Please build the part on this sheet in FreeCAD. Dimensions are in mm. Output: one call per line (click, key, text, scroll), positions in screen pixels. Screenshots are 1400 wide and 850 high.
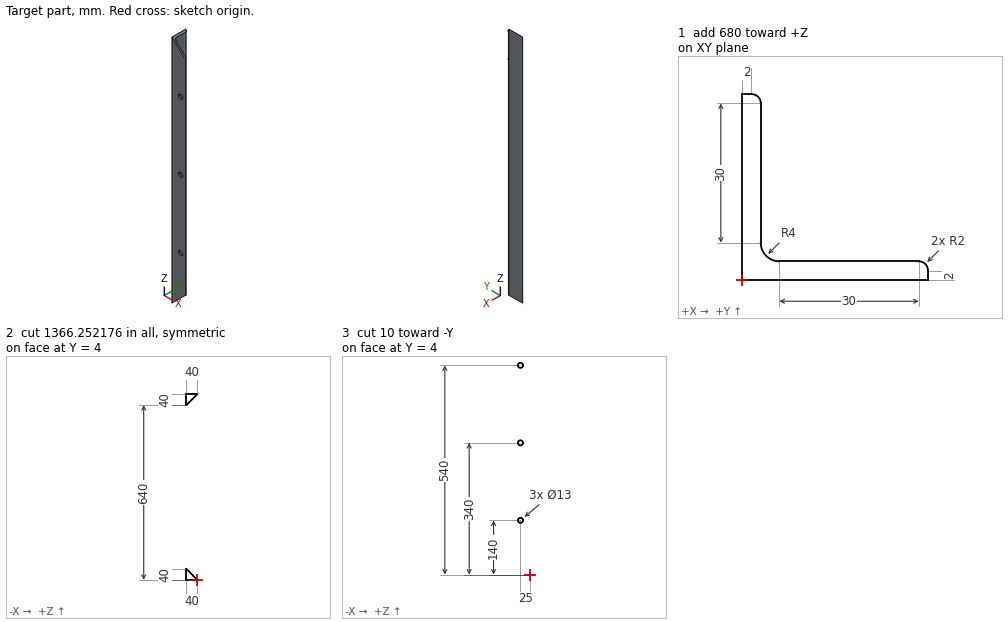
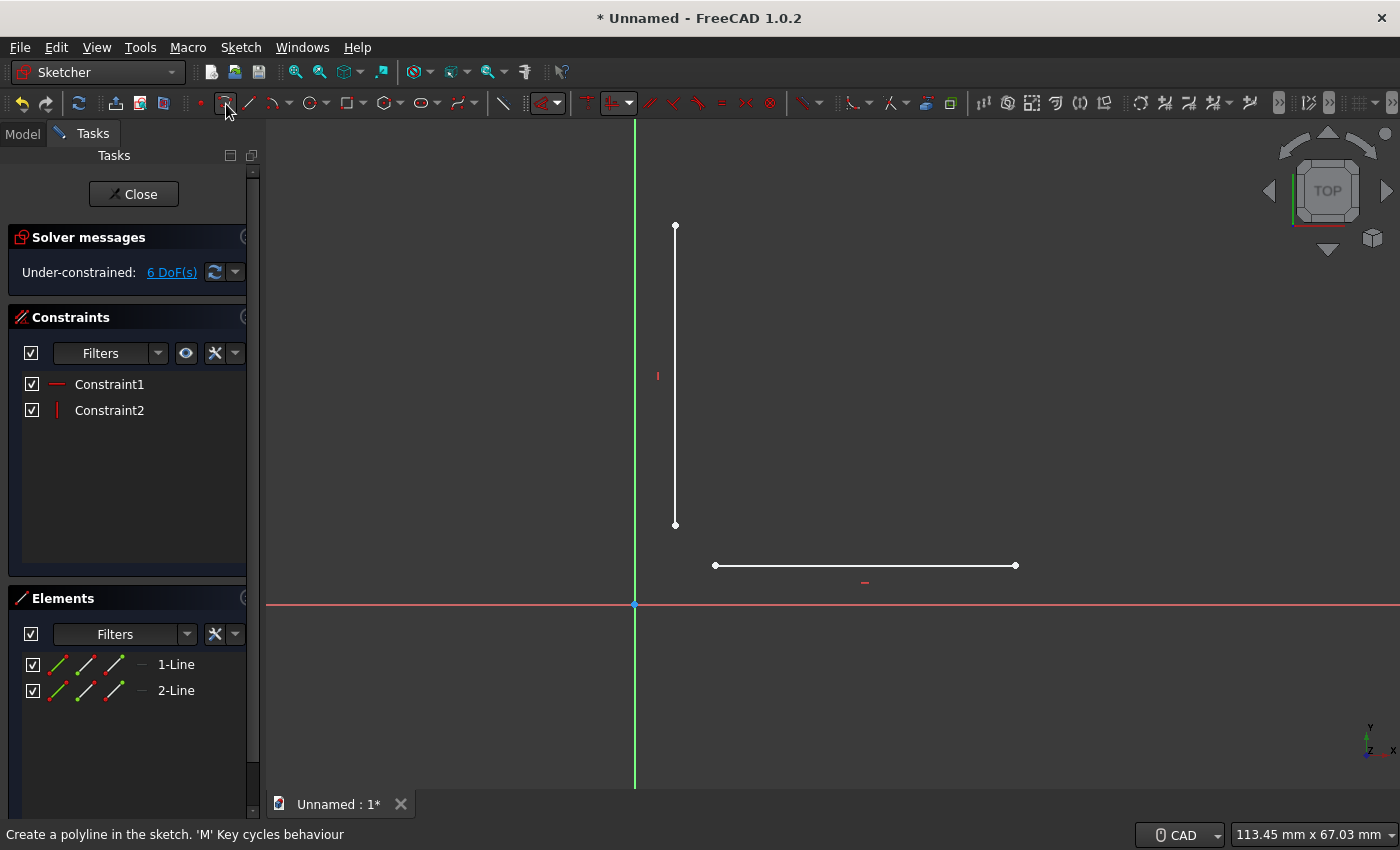
click(655, 205)
click(635, 205)
click(635, 605)
click(1035, 596)
click(1035, 585)
right_click(1035, 585)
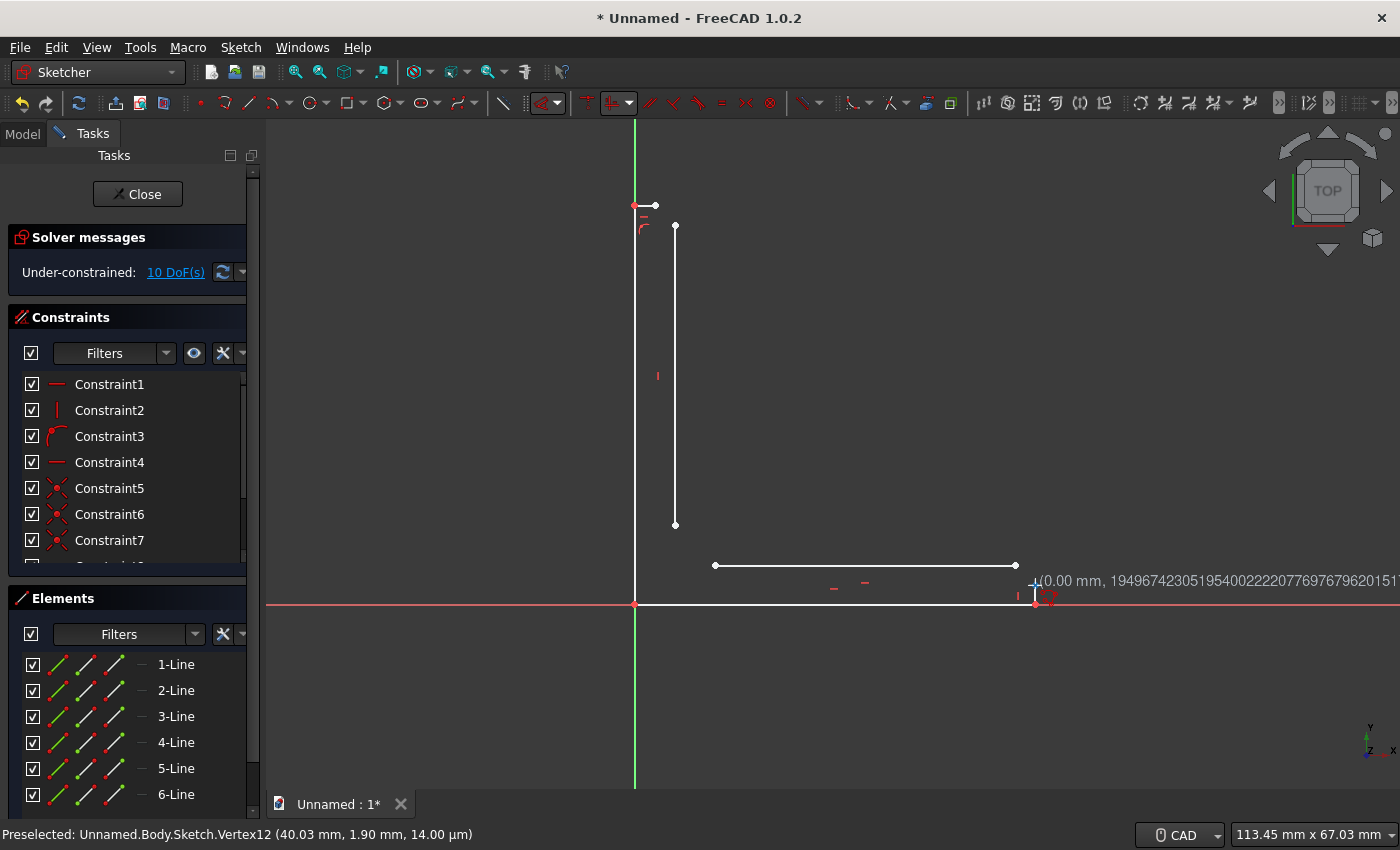
key(g)
key(3)
key(a)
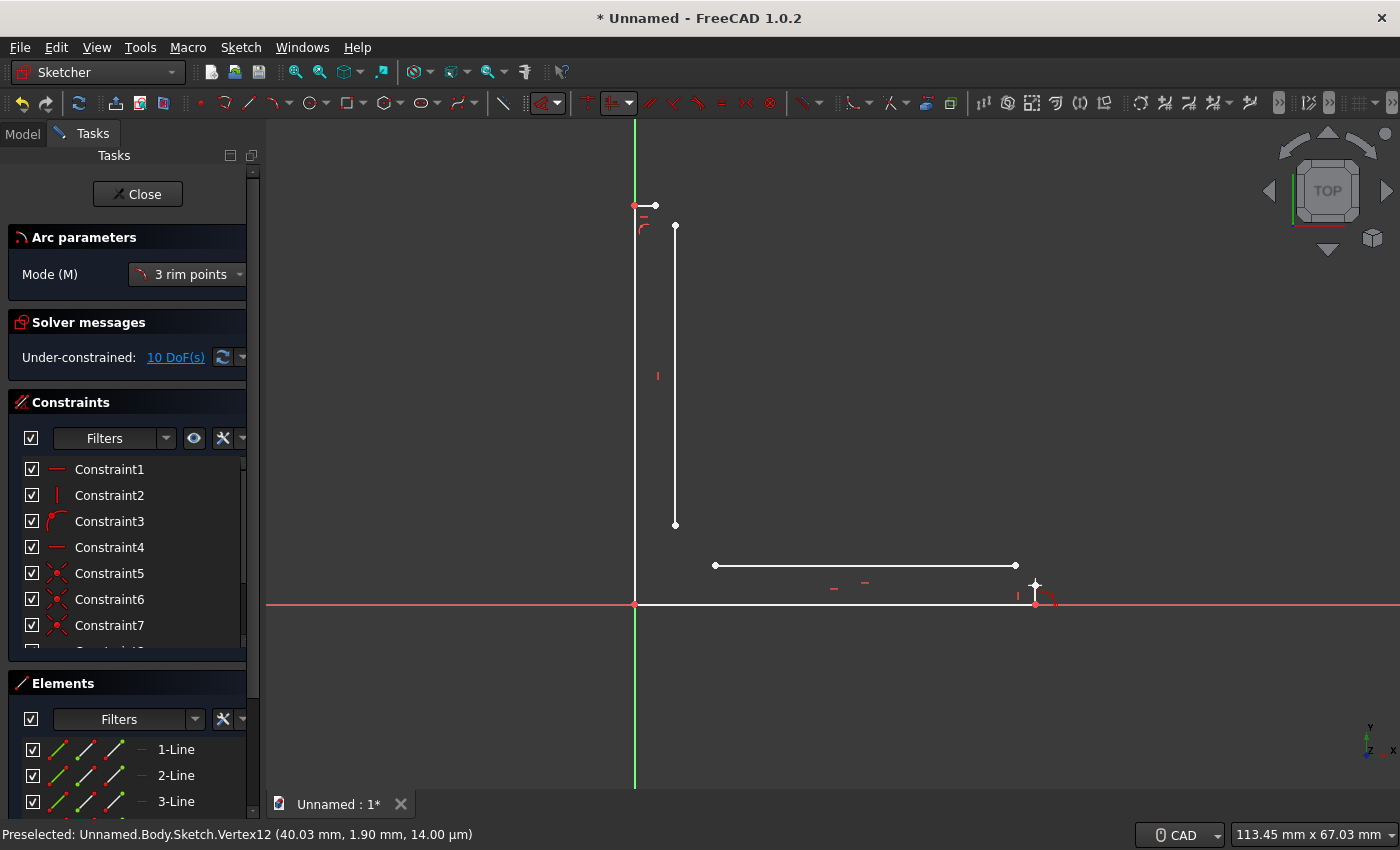
click(715, 566)
click(675, 526)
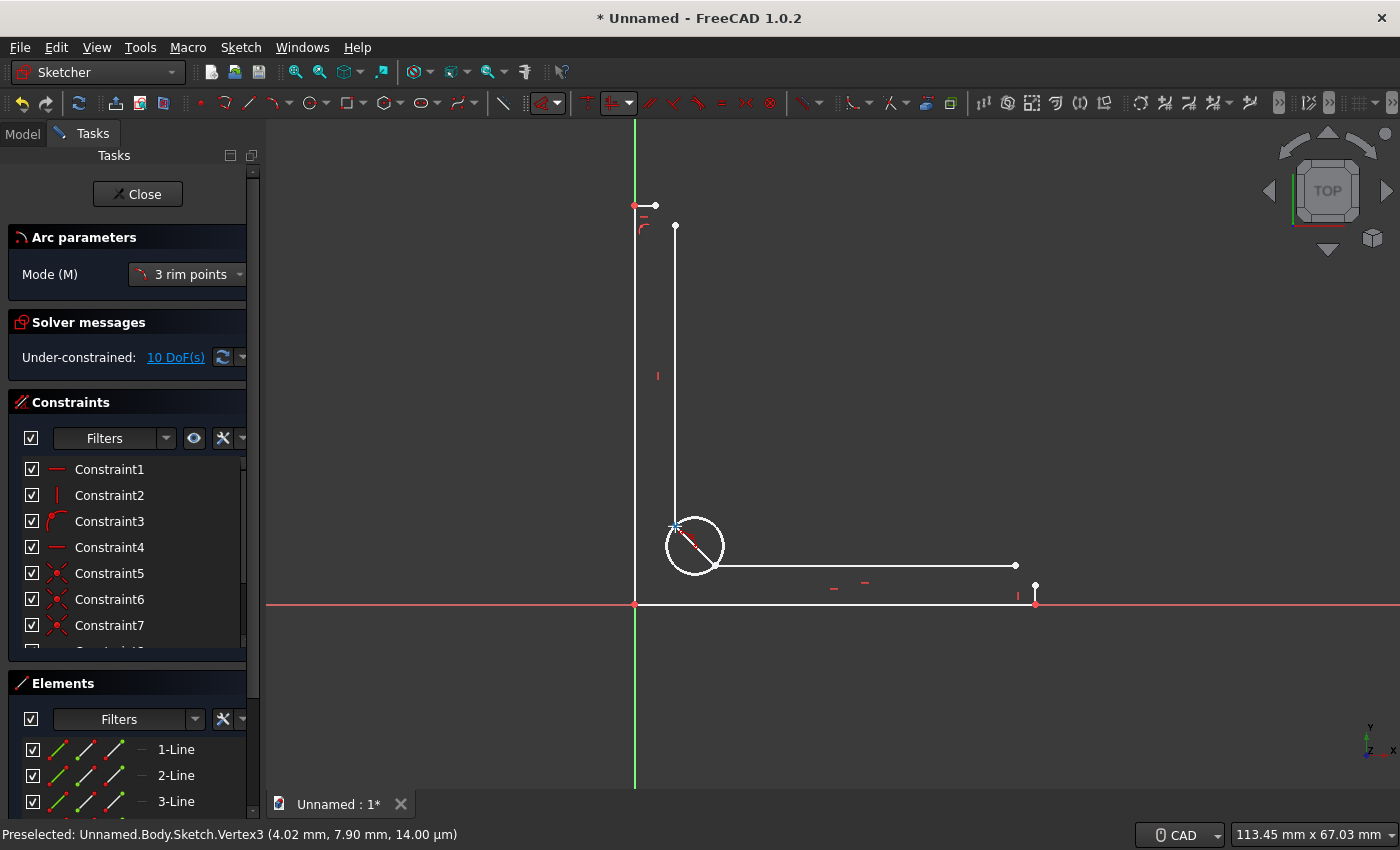
scroll(687, 553, up, 2)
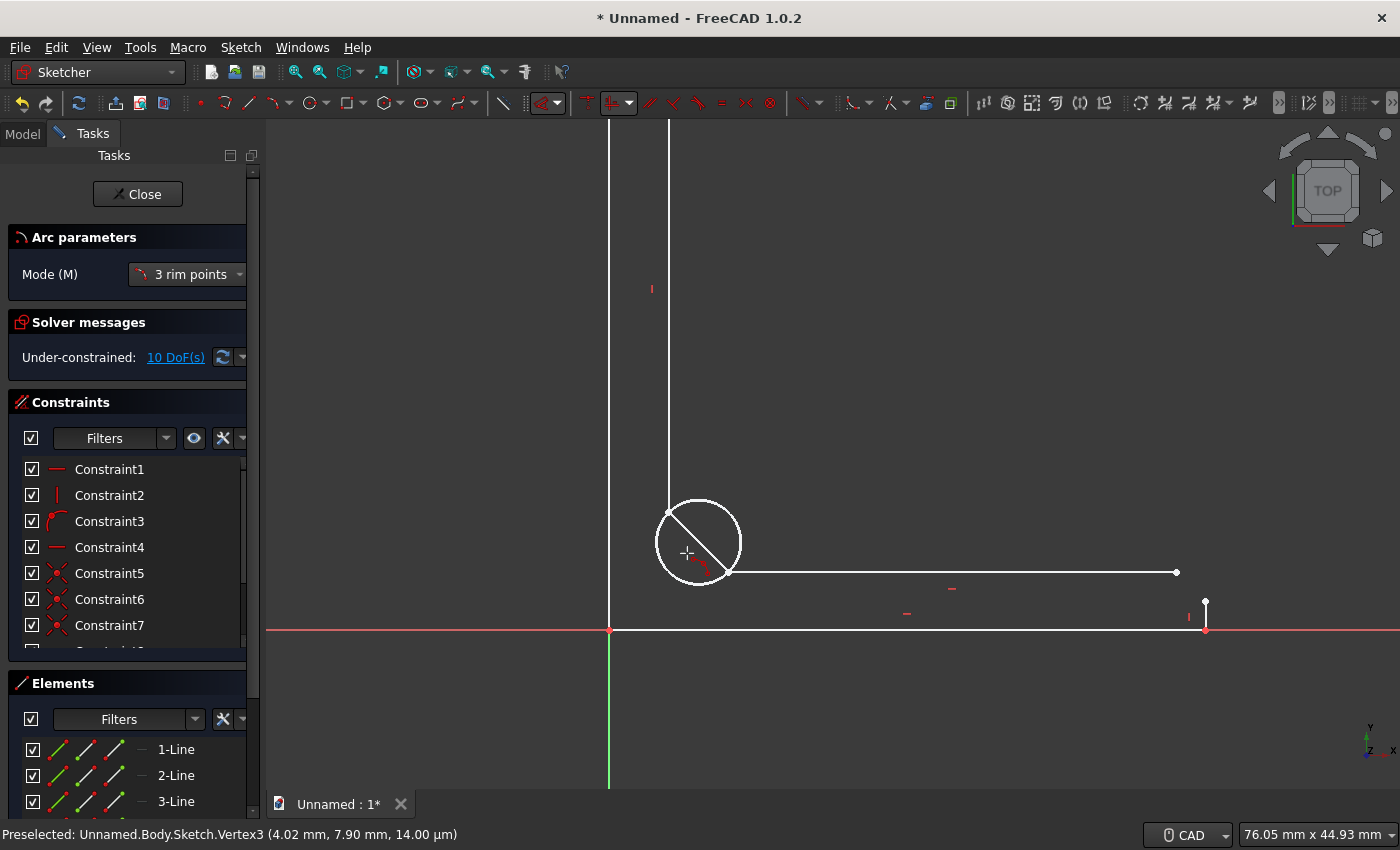
click(686, 553)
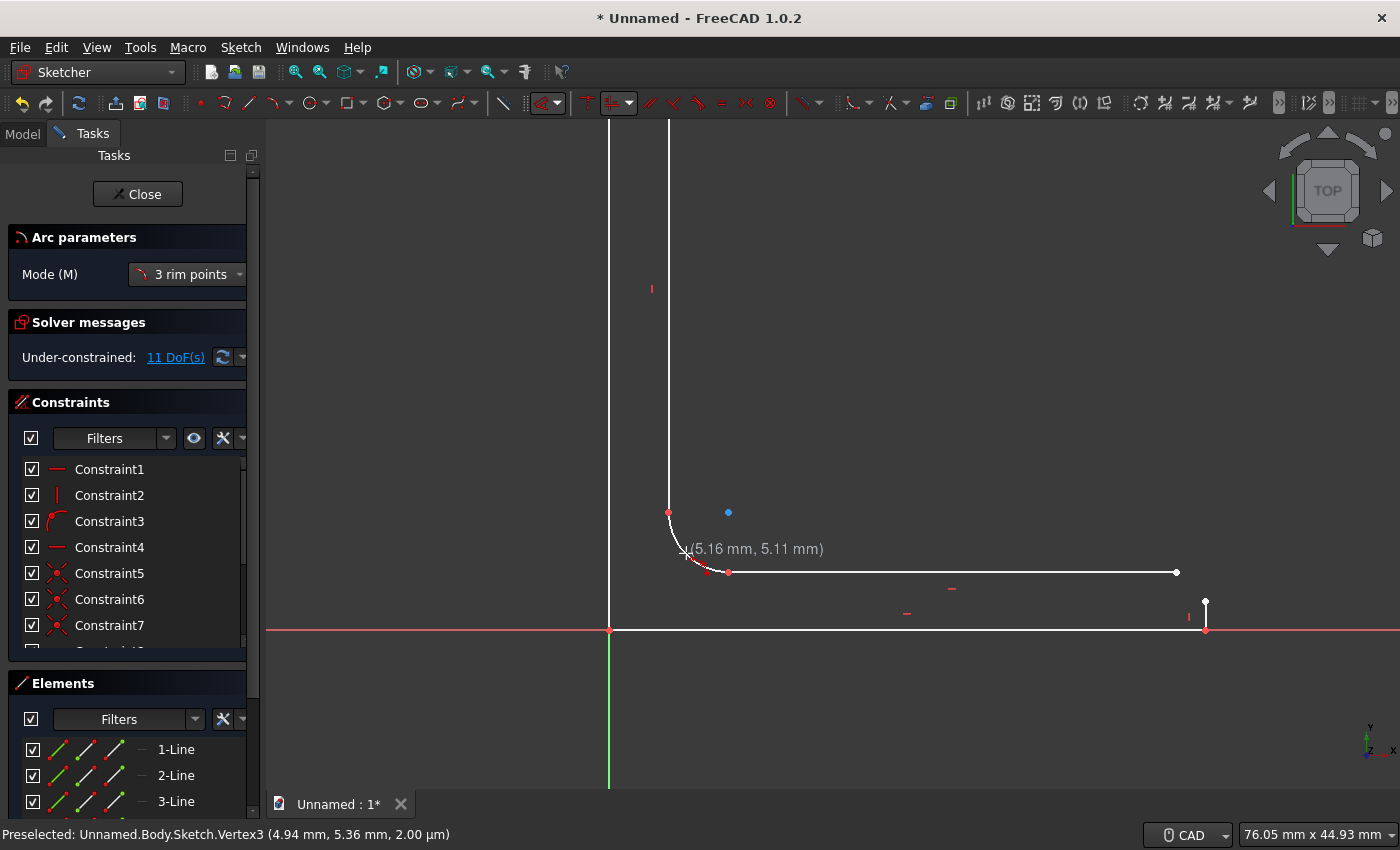
scroll(474, 702, down, 2)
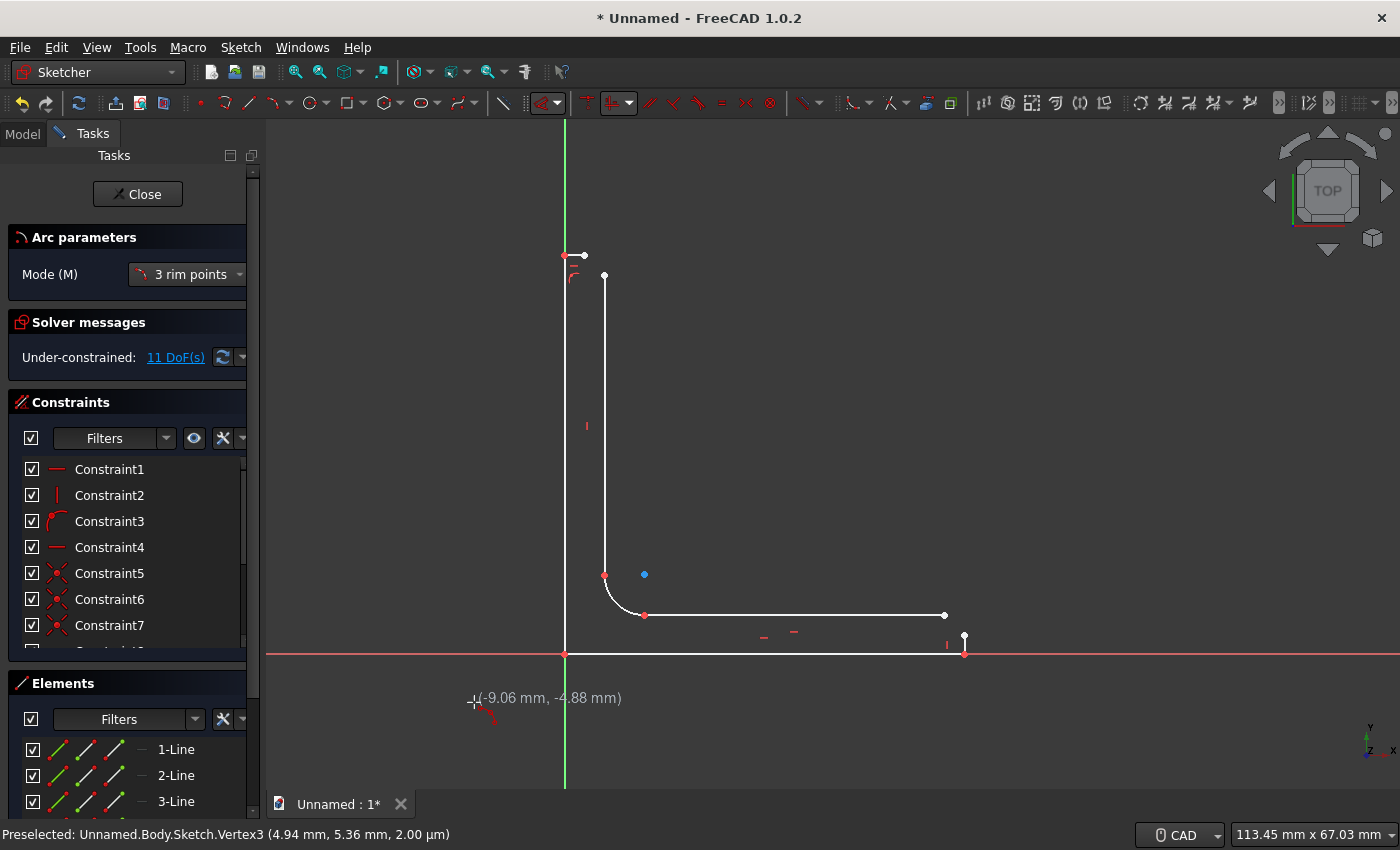
click(605, 275)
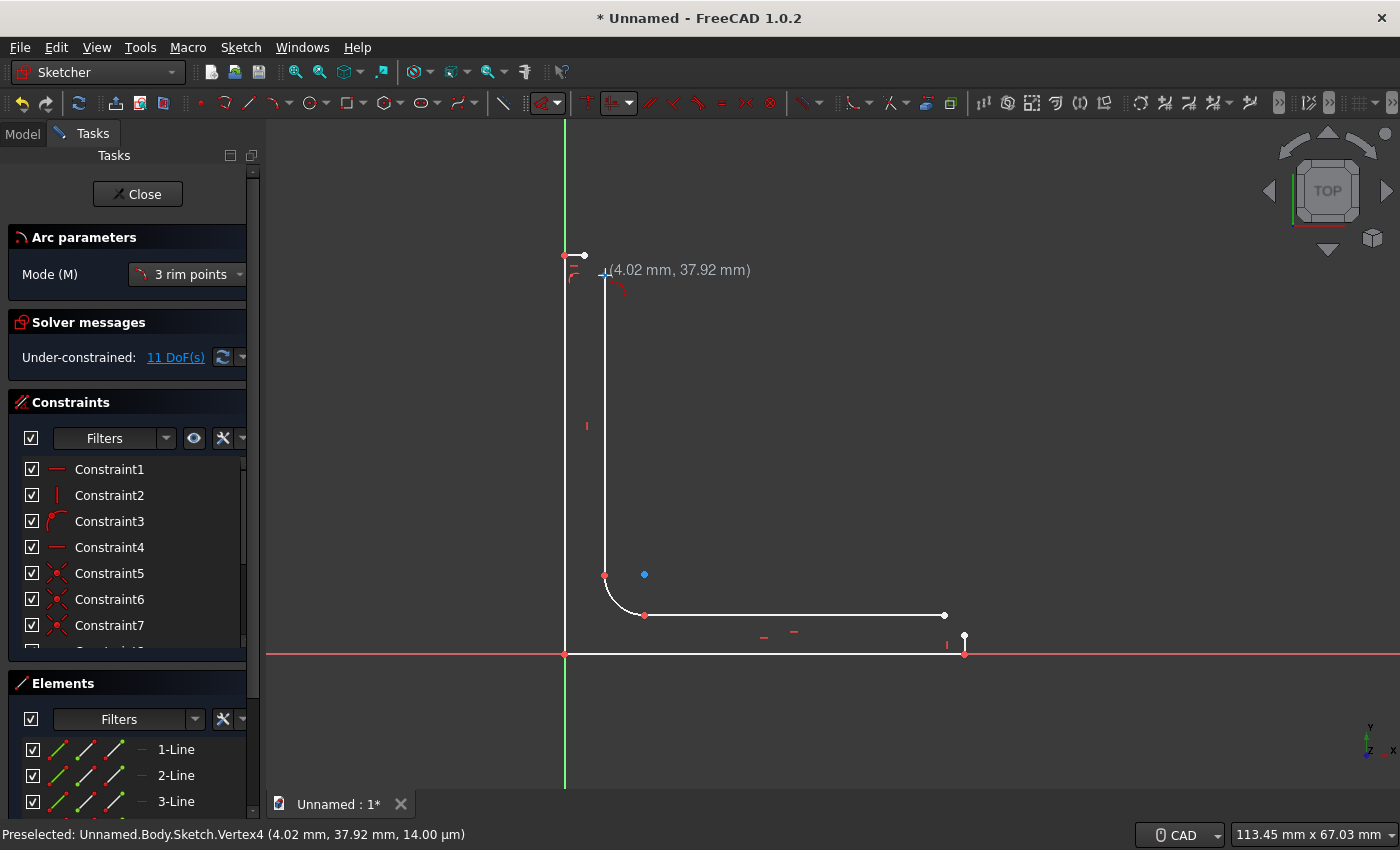
scroll(585, 254, up, 3)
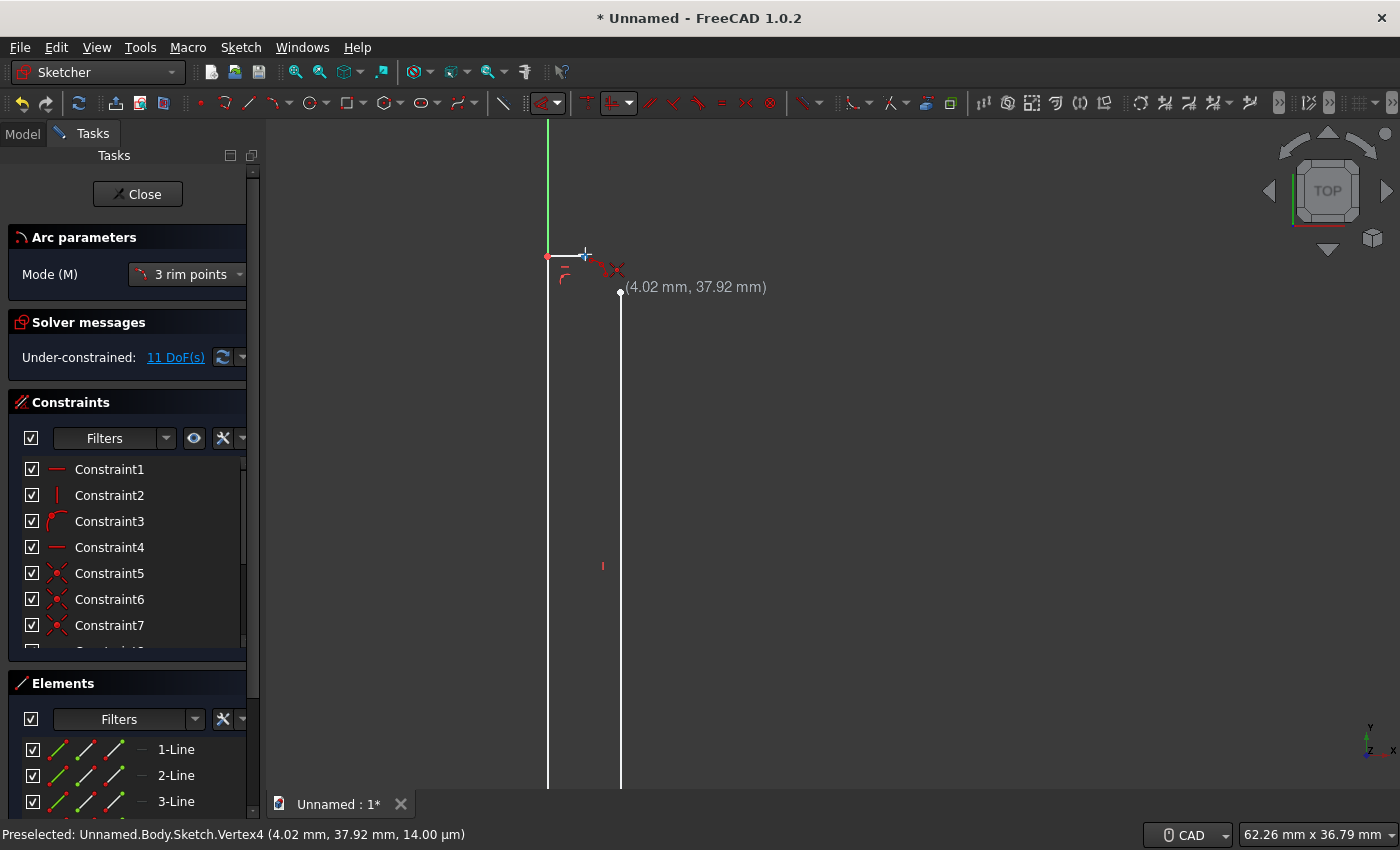
click(584, 256)